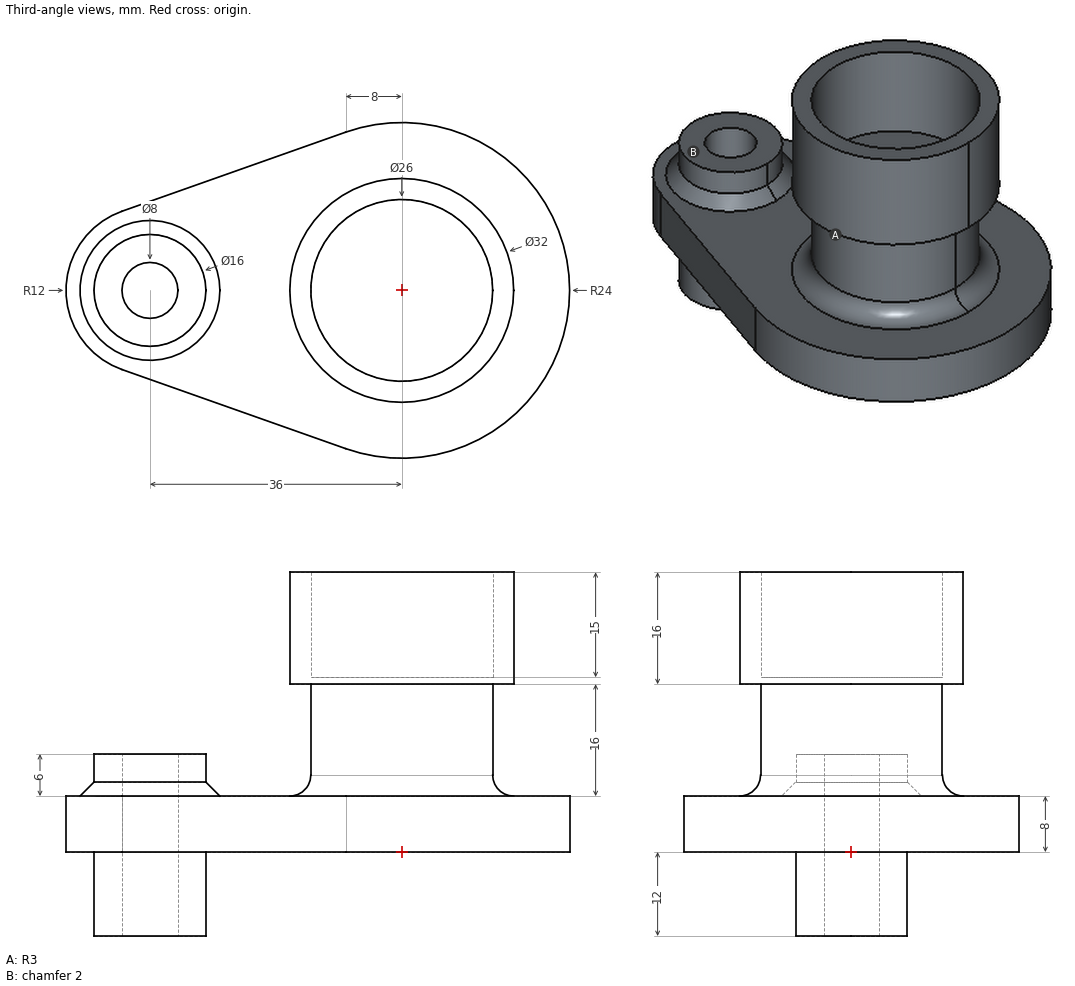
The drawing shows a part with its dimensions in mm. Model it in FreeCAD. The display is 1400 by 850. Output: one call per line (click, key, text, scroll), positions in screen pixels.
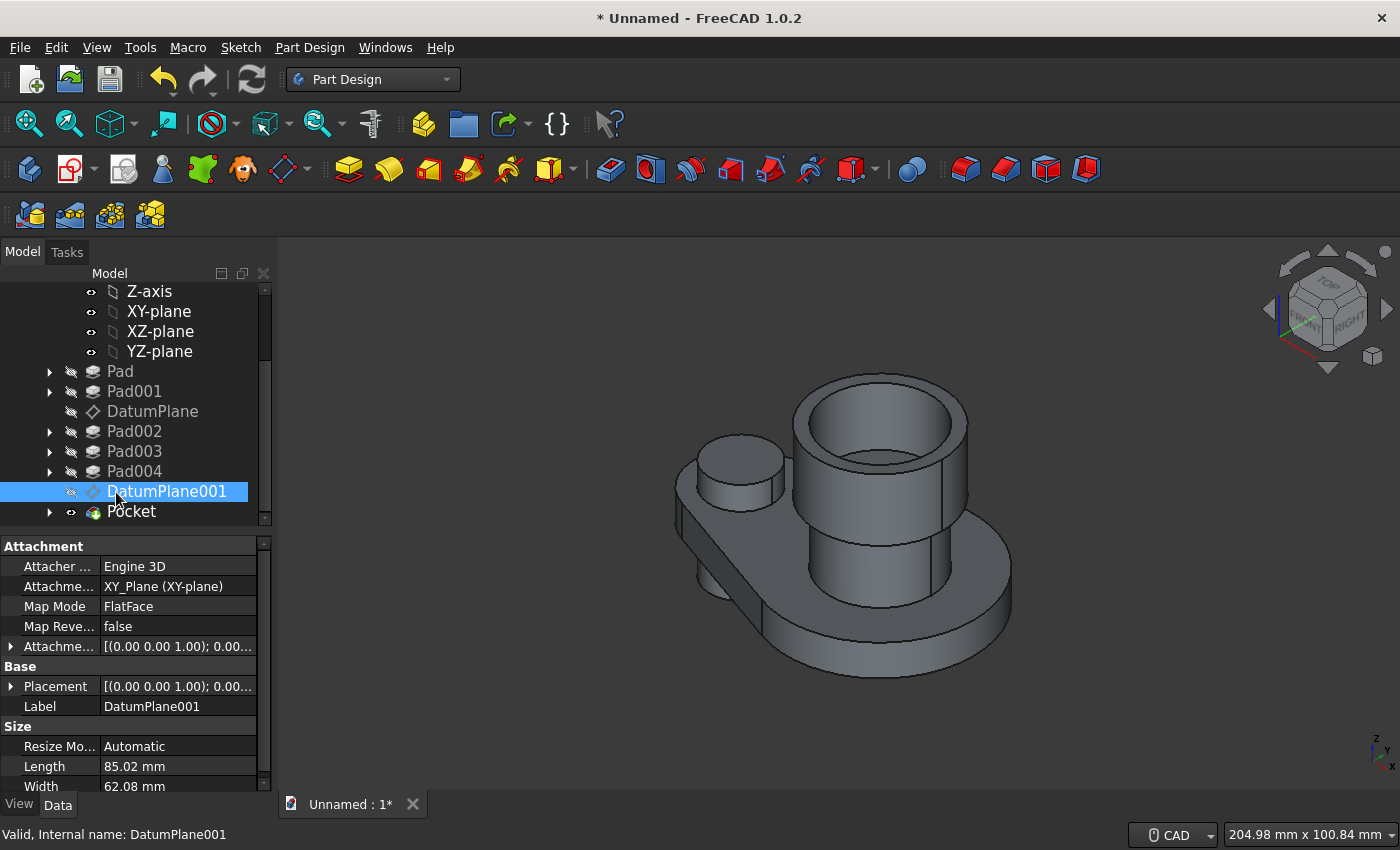
key(2)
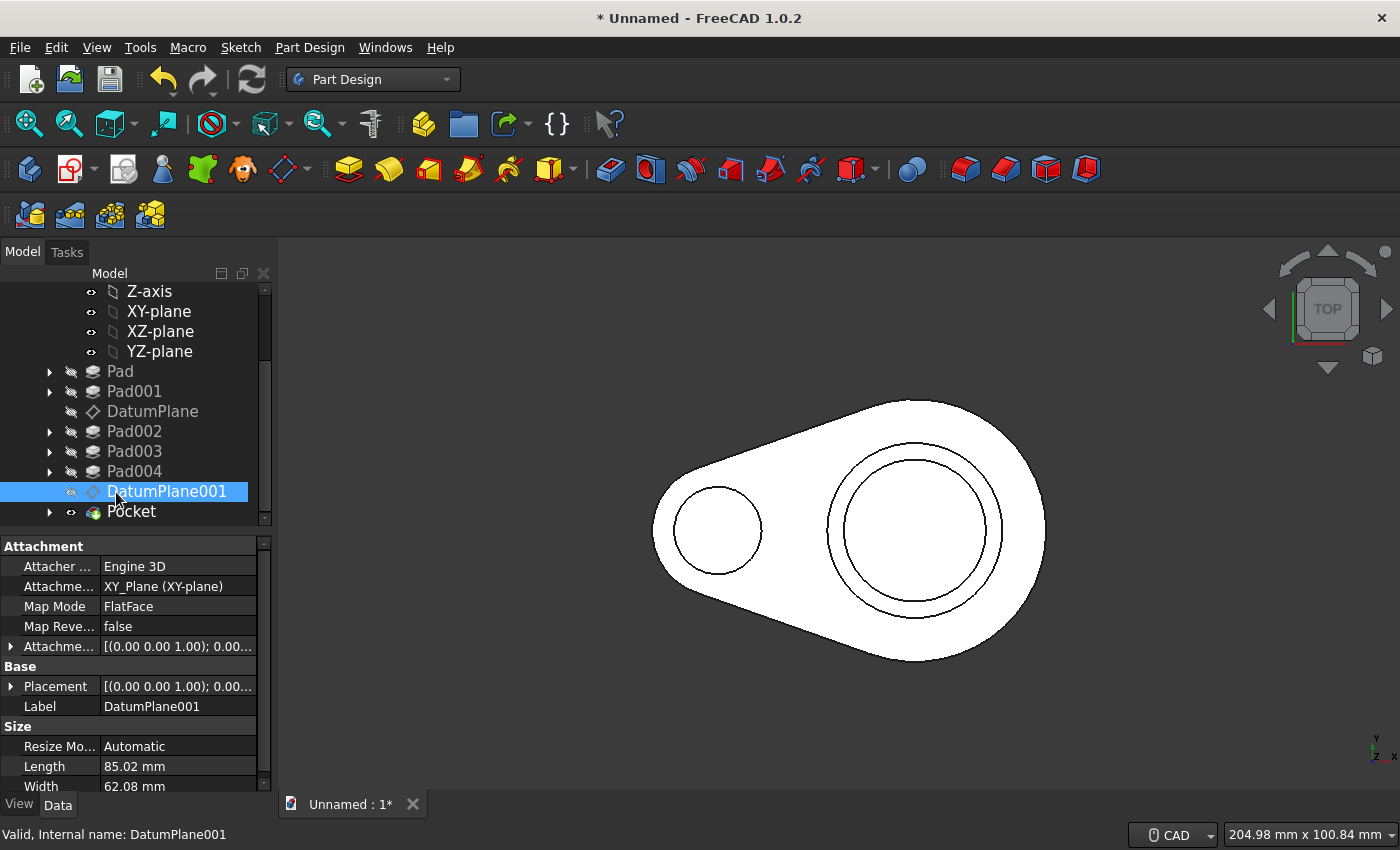
key(1)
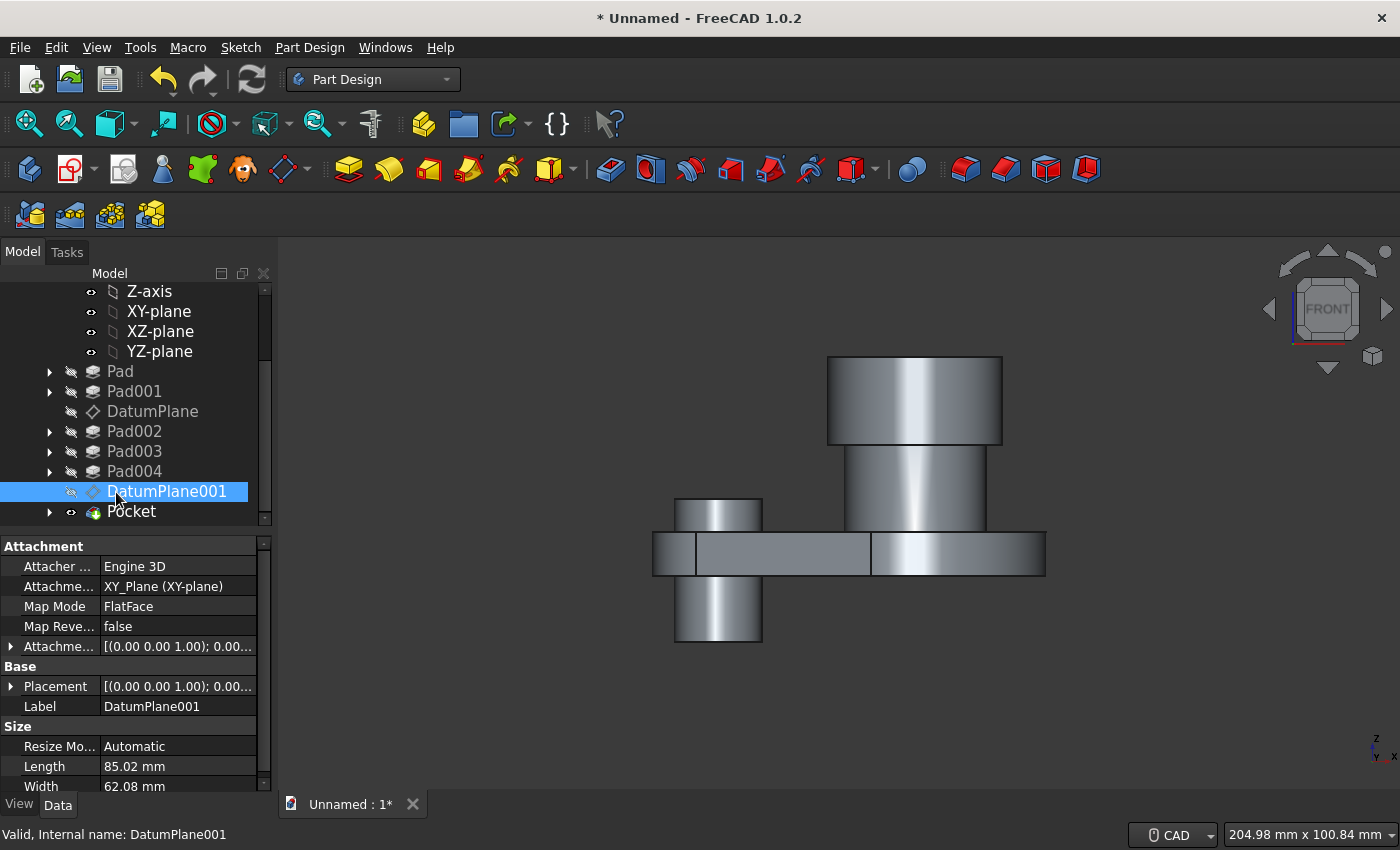
key(3)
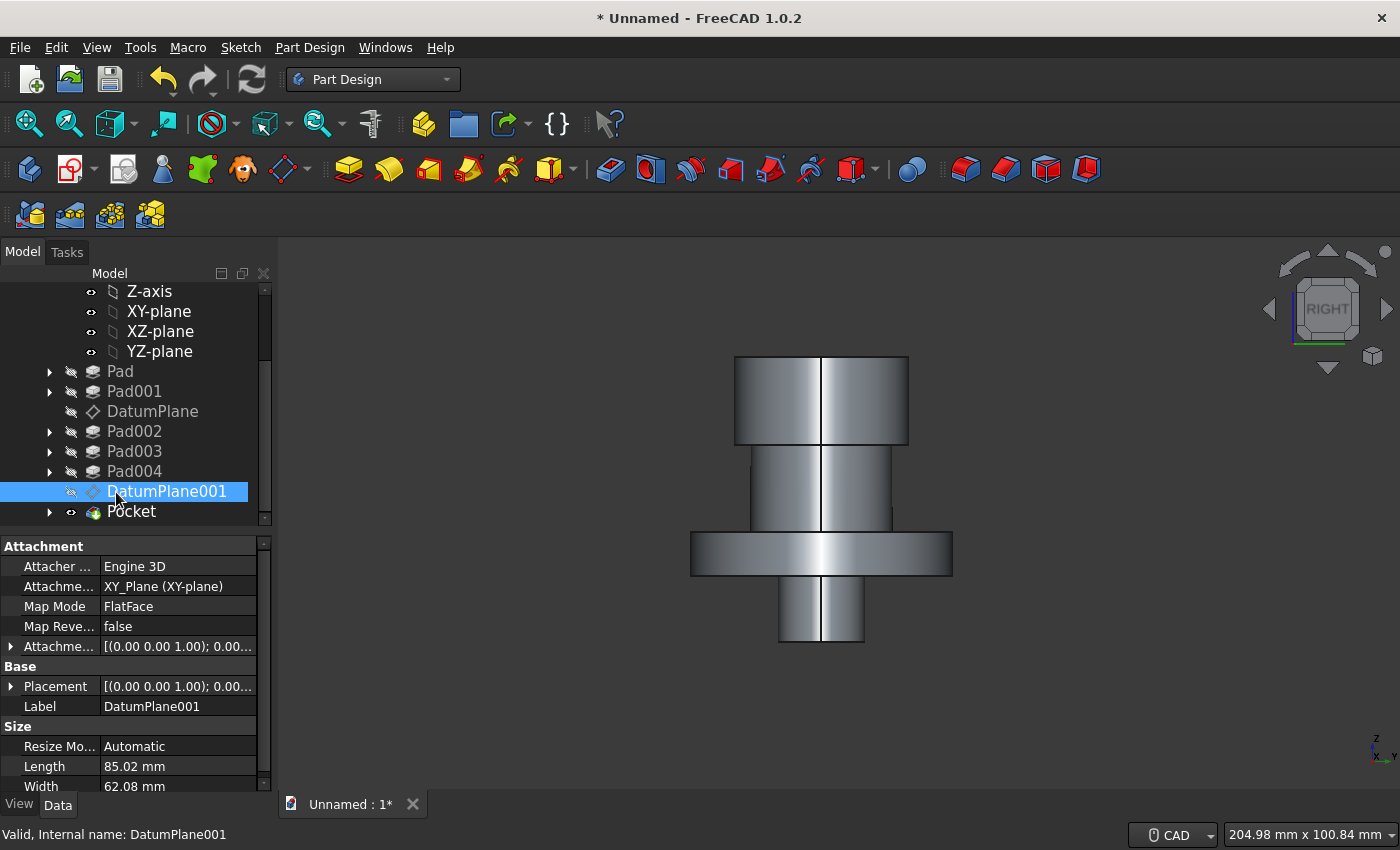
key(5)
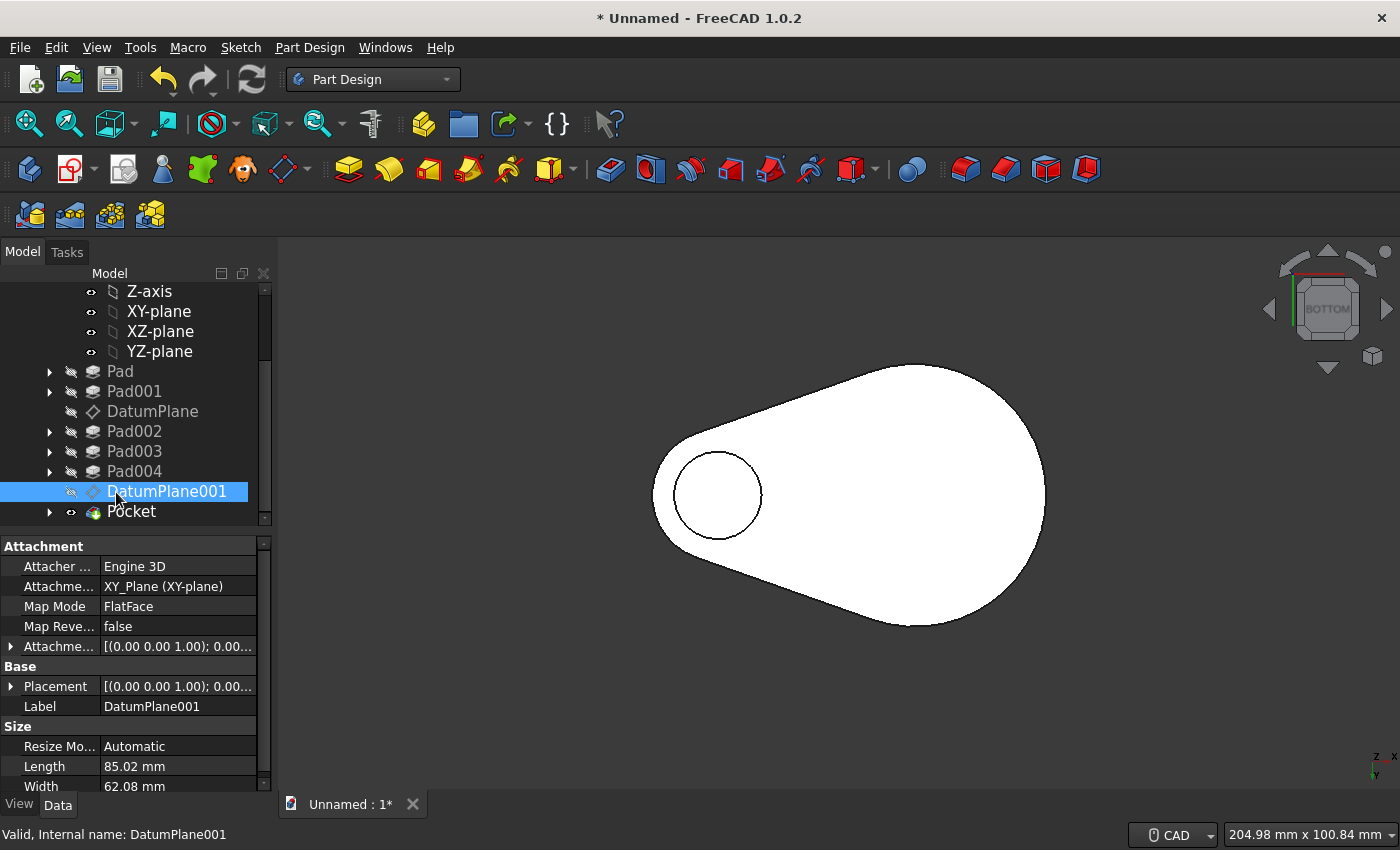
key(4)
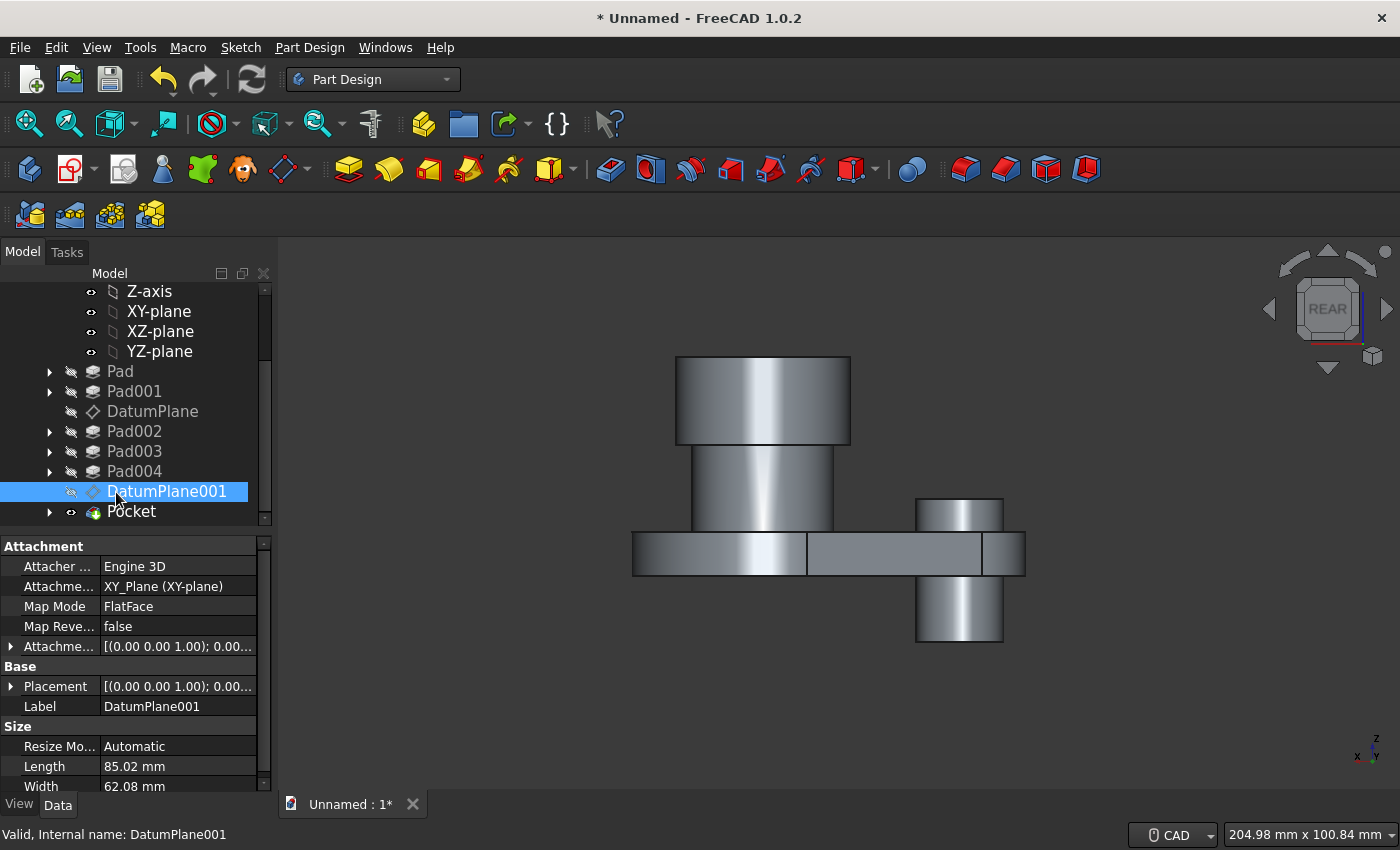
key(6)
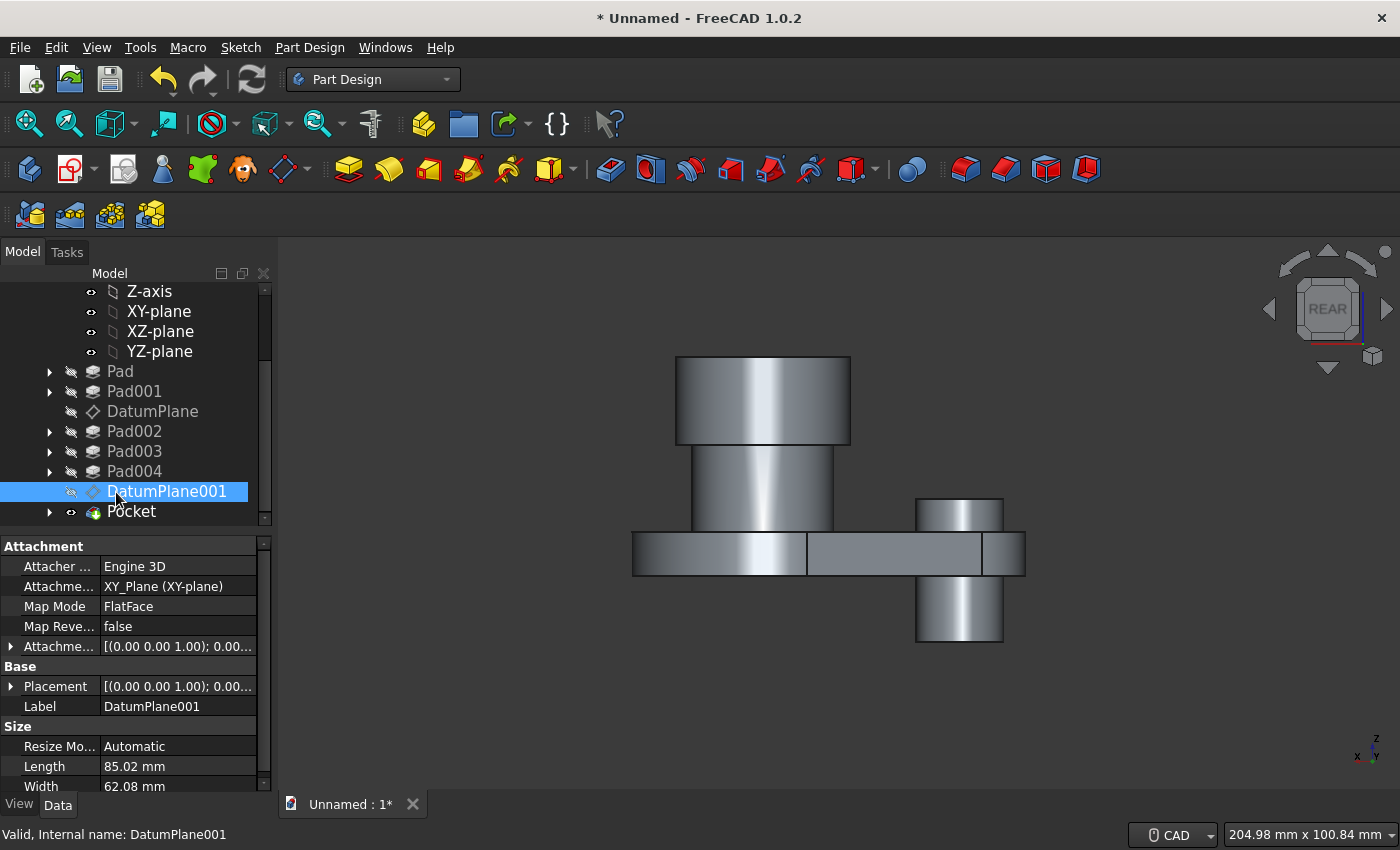
key(v)
key(3)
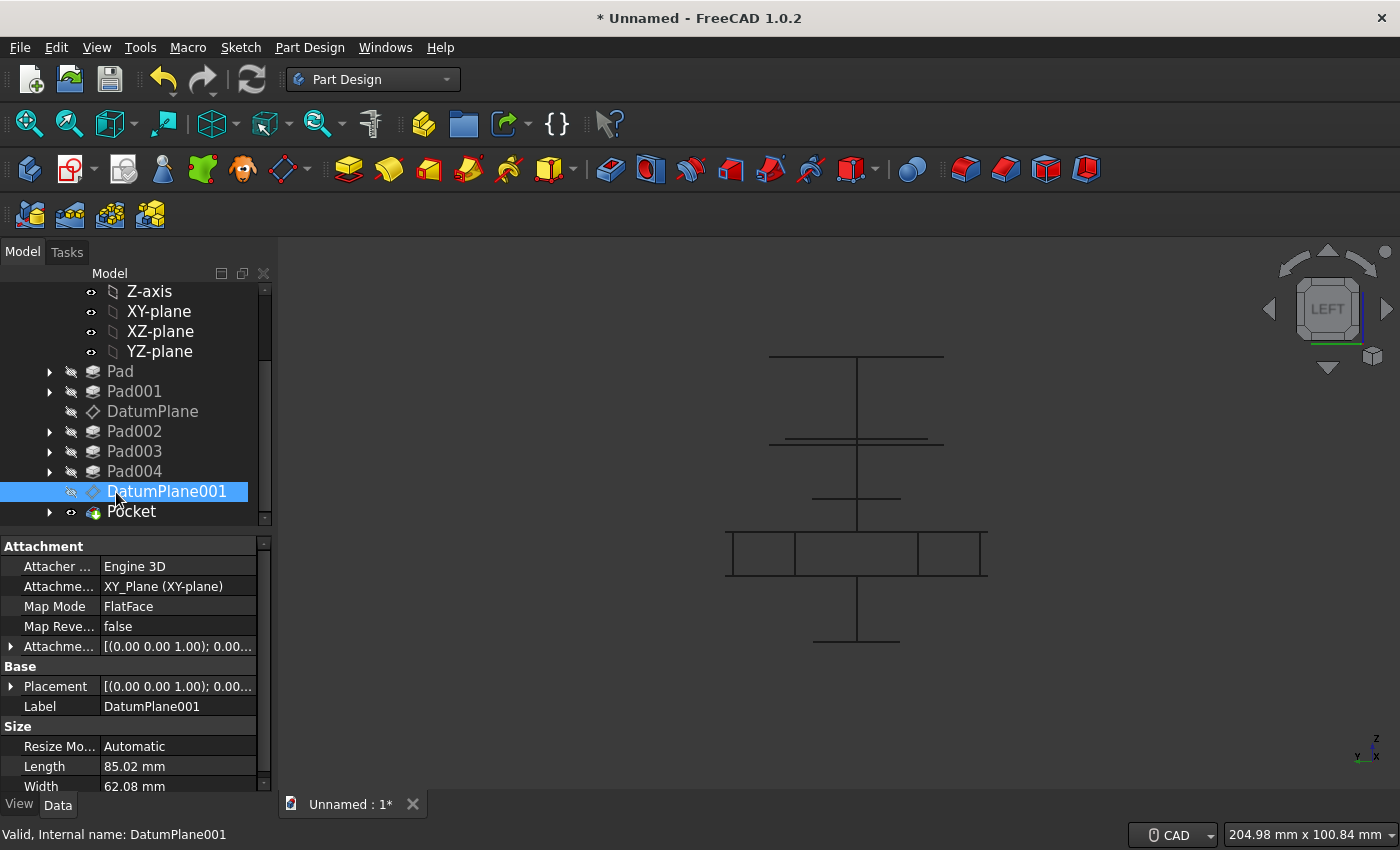
key(0)